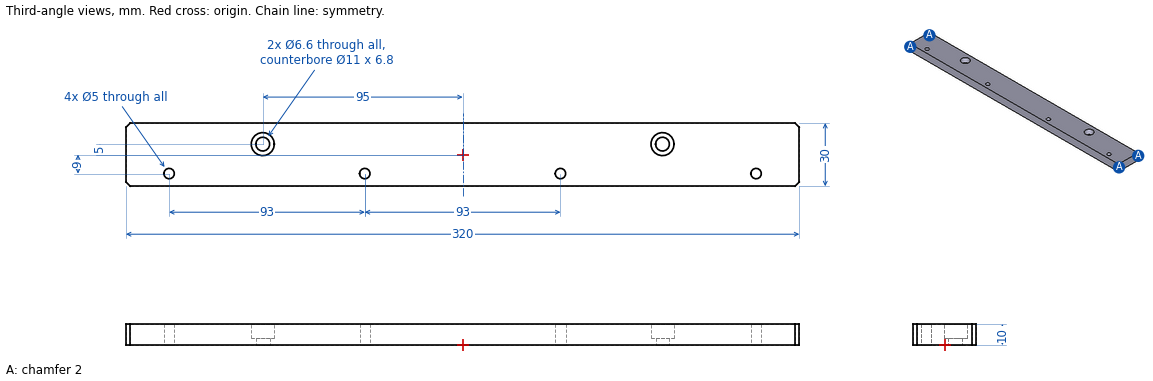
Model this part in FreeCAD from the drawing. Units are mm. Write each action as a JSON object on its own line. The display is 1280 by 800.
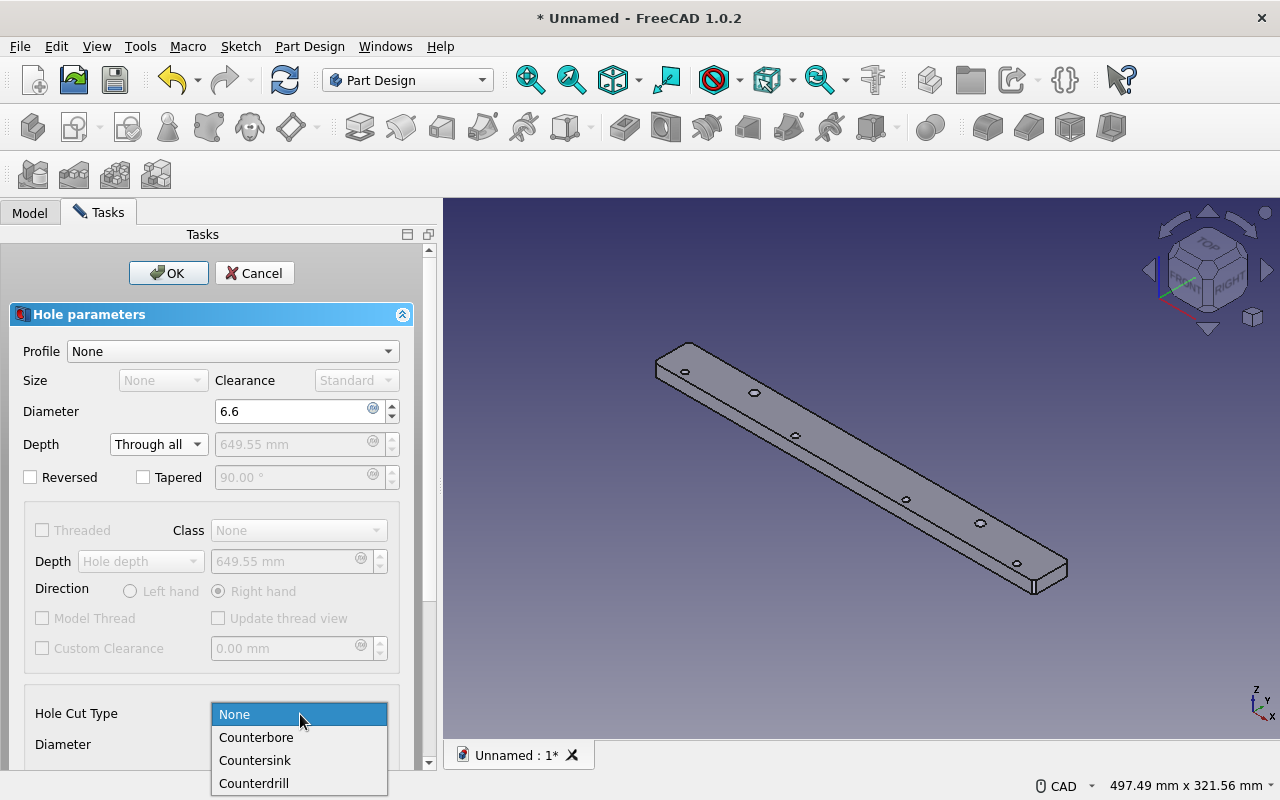
{"action": "left_click", "coordinate": [298, 738]}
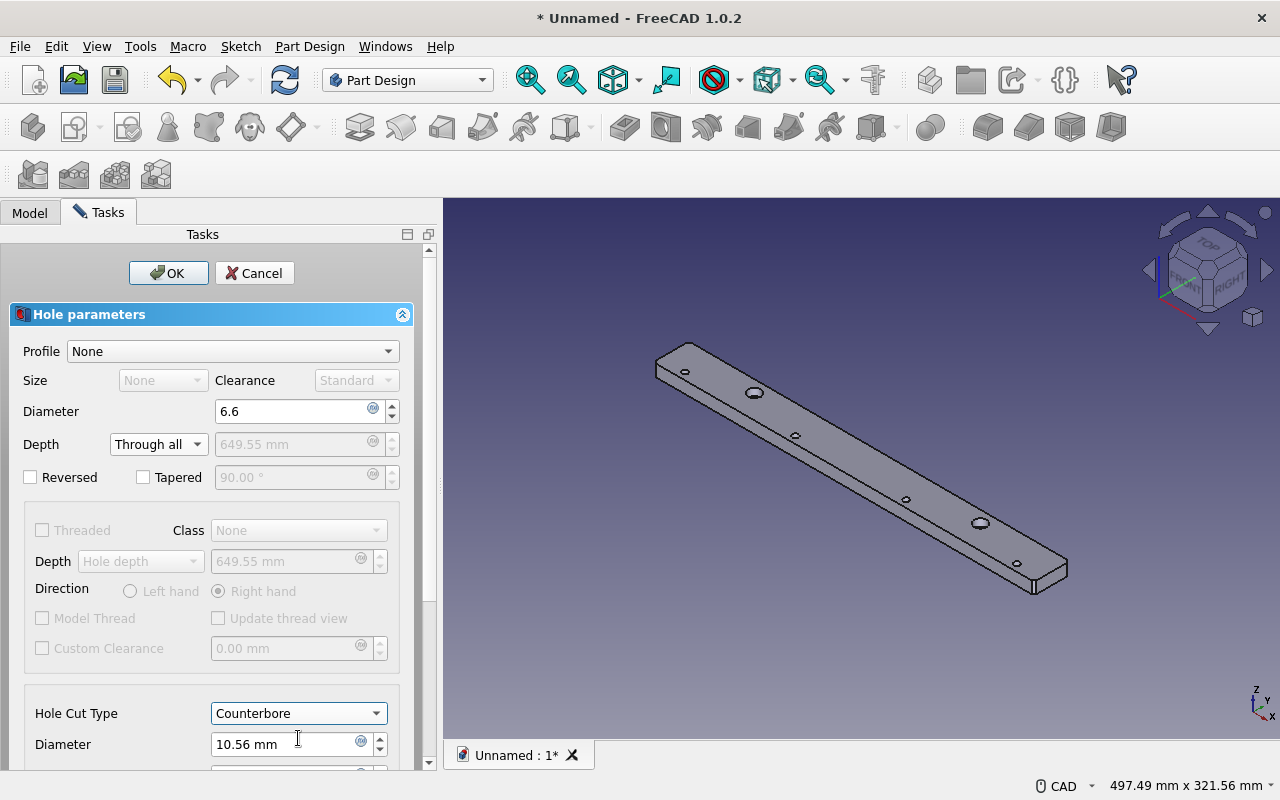
{"action": "triple_click", "coordinate": [292, 744]}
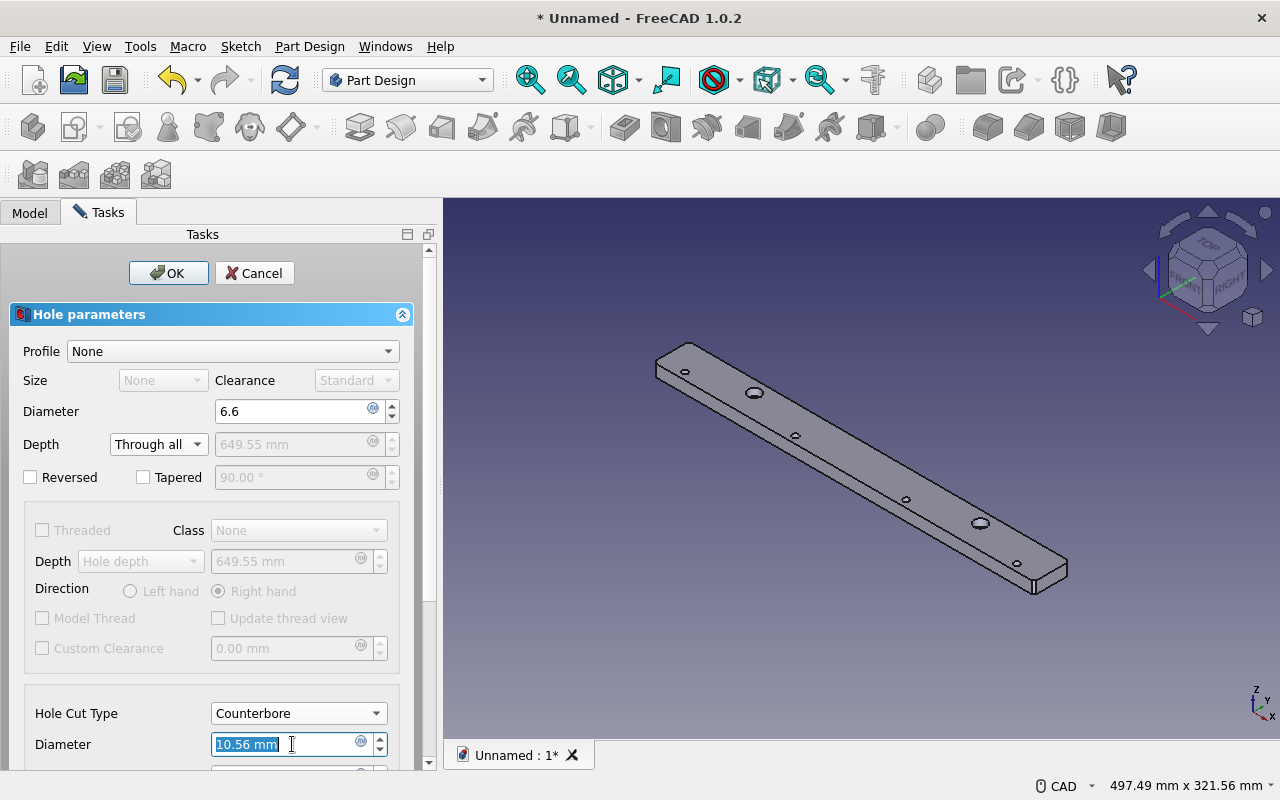
{"action": "type", "text": "11"}
{"action": "key", "text": "Tab"}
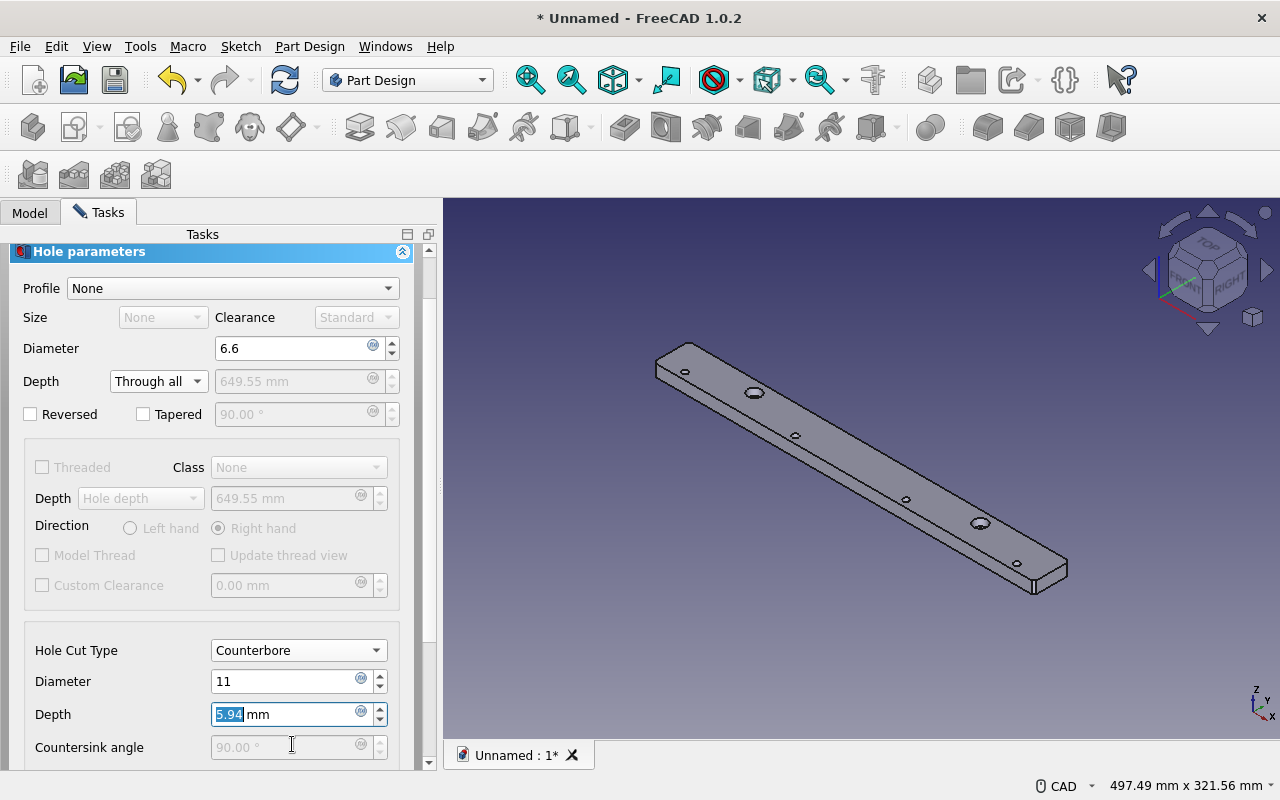
{"action": "type", "text": "6.8"}
{"action": "key", "text": "Tab"}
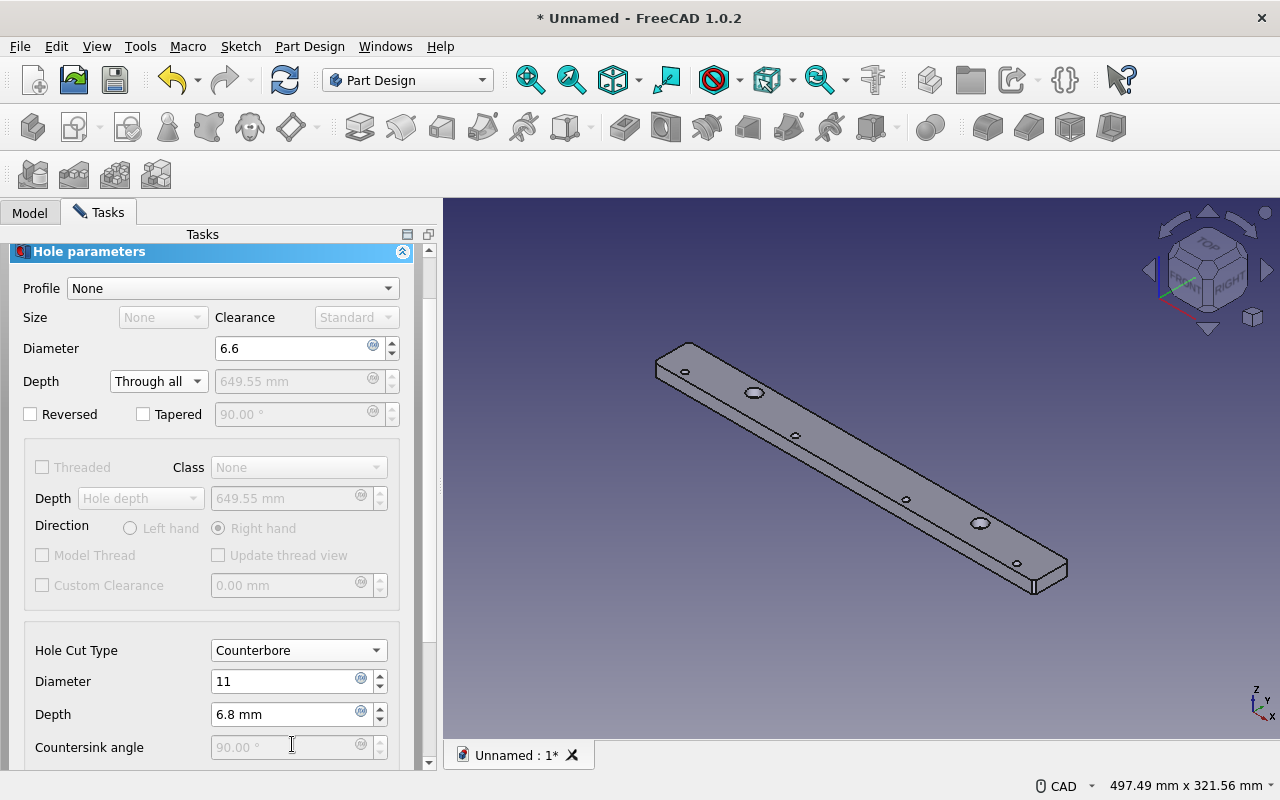
{"action": "scroll", "coordinate": [429, 507], "scroll_direction": "up", "scroll_amount": 2}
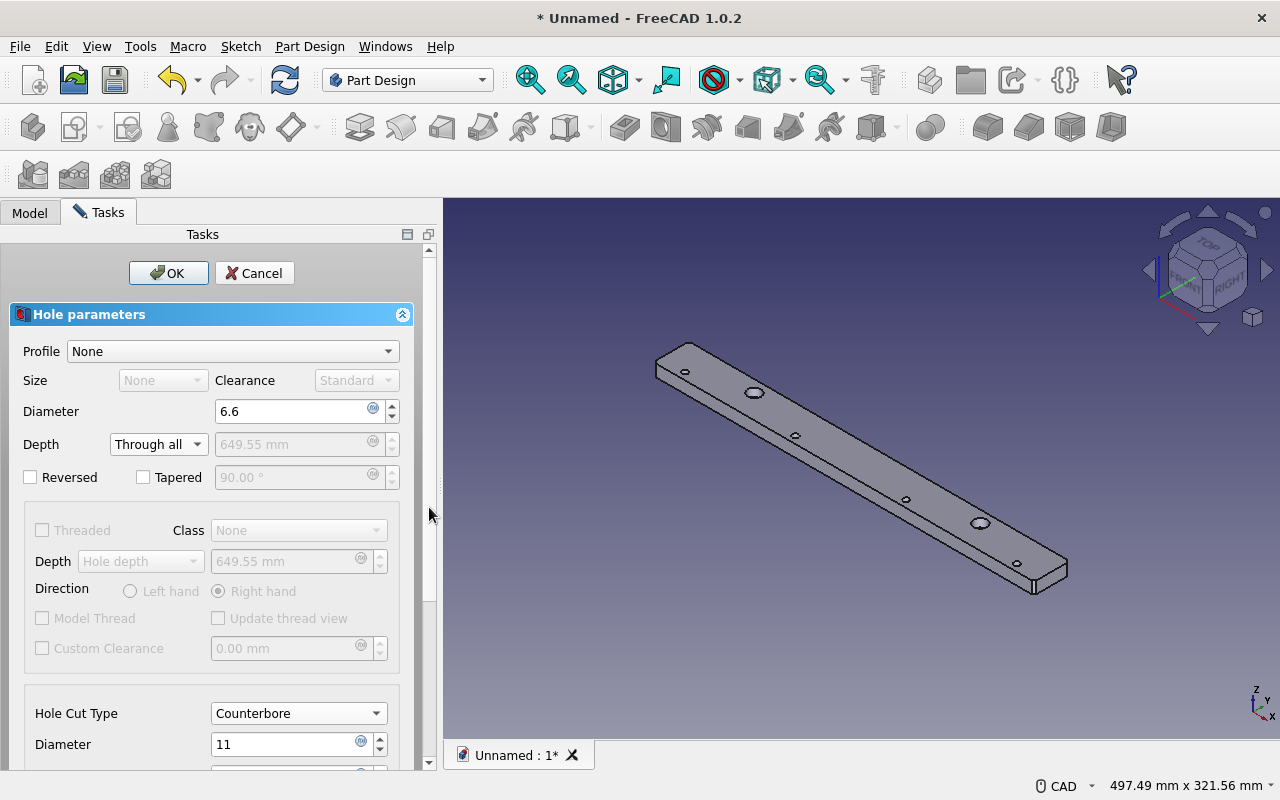
{"action": "left_click", "coordinate": [169, 273]}